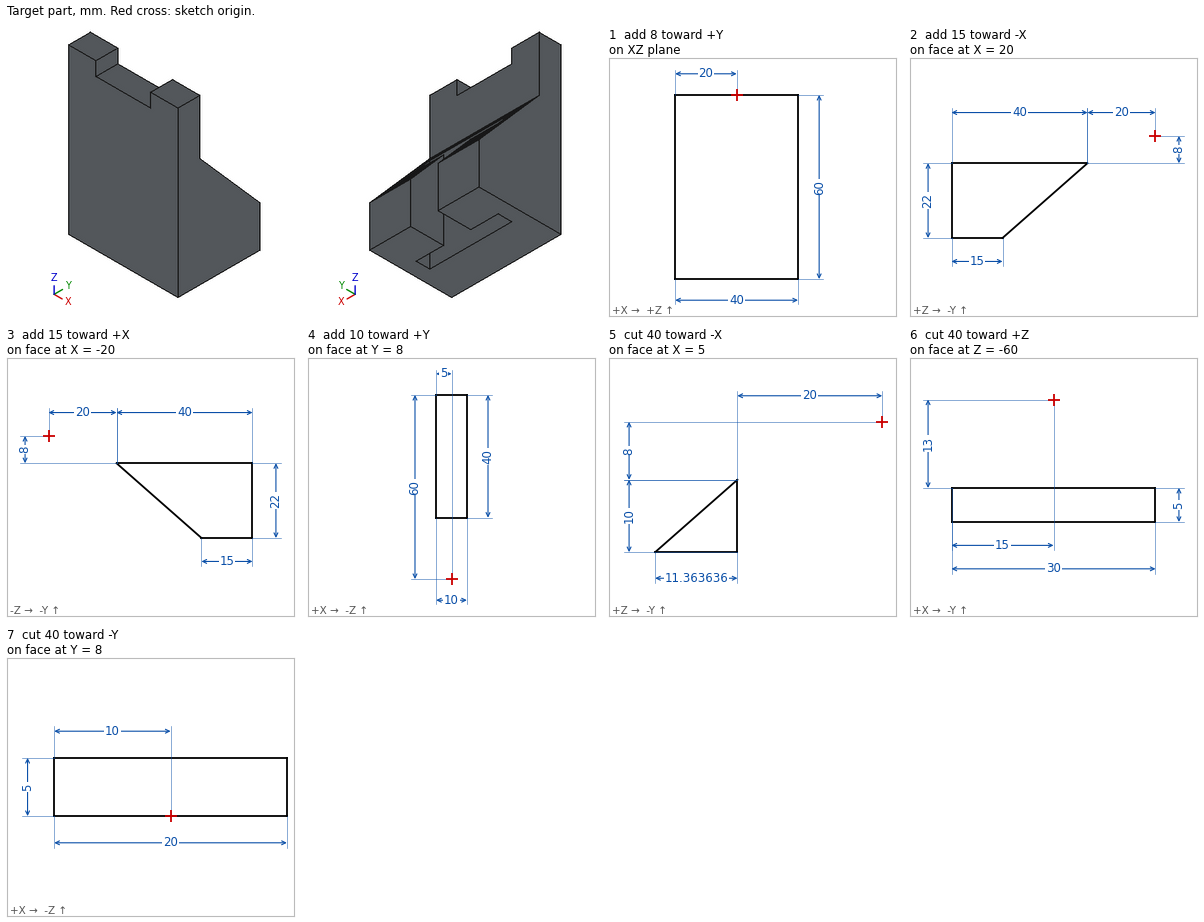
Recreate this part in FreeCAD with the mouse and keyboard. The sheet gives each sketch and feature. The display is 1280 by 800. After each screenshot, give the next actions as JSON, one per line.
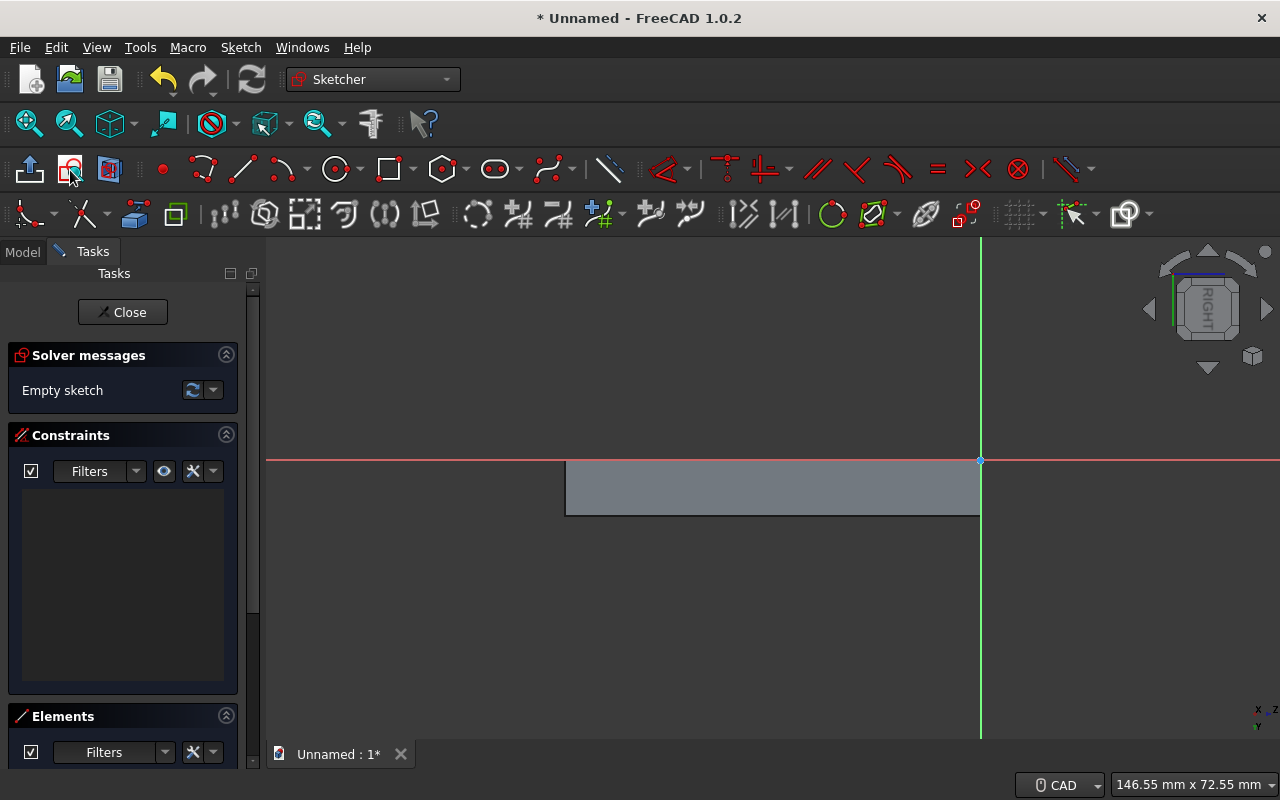
{"action": "scroll", "coordinate": [912, 711], "scroll_direction": "up", "scroll_amount": 2}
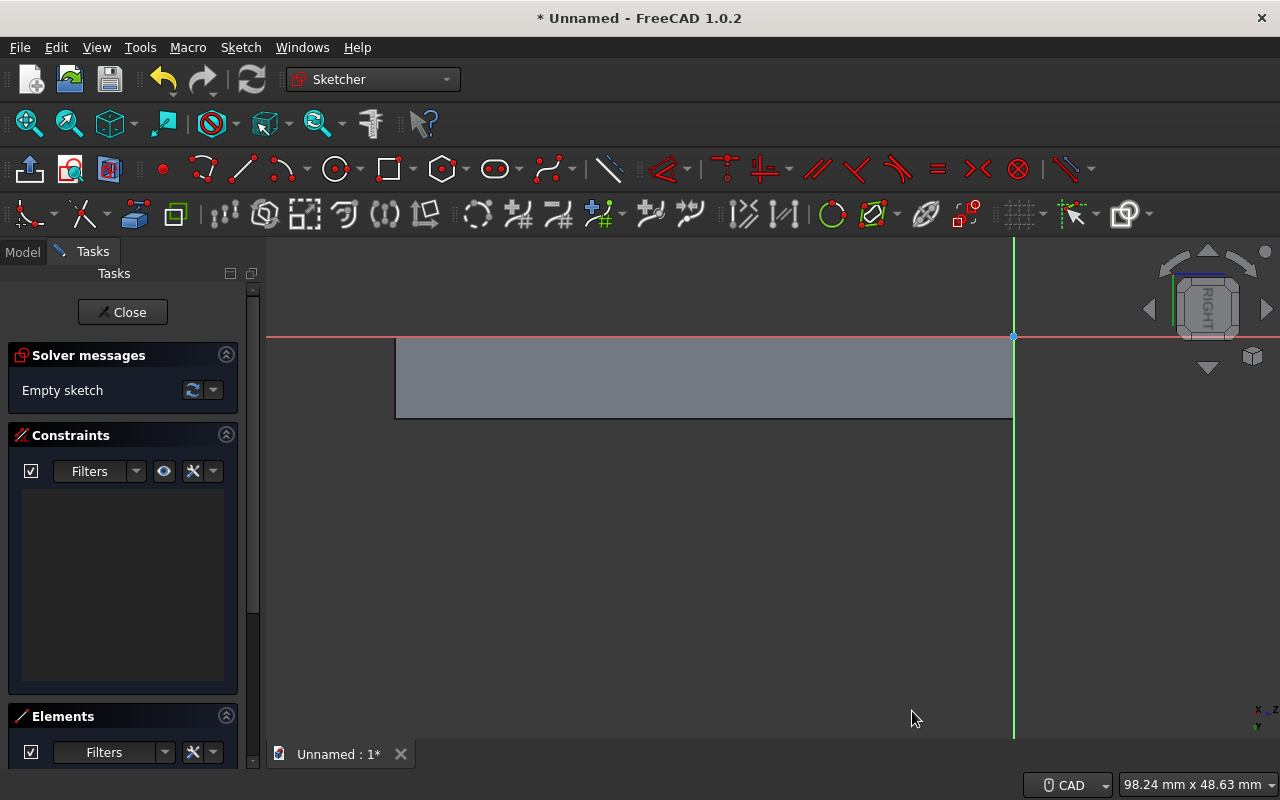
{"action": "left_click", "coordinate": [204, 170]}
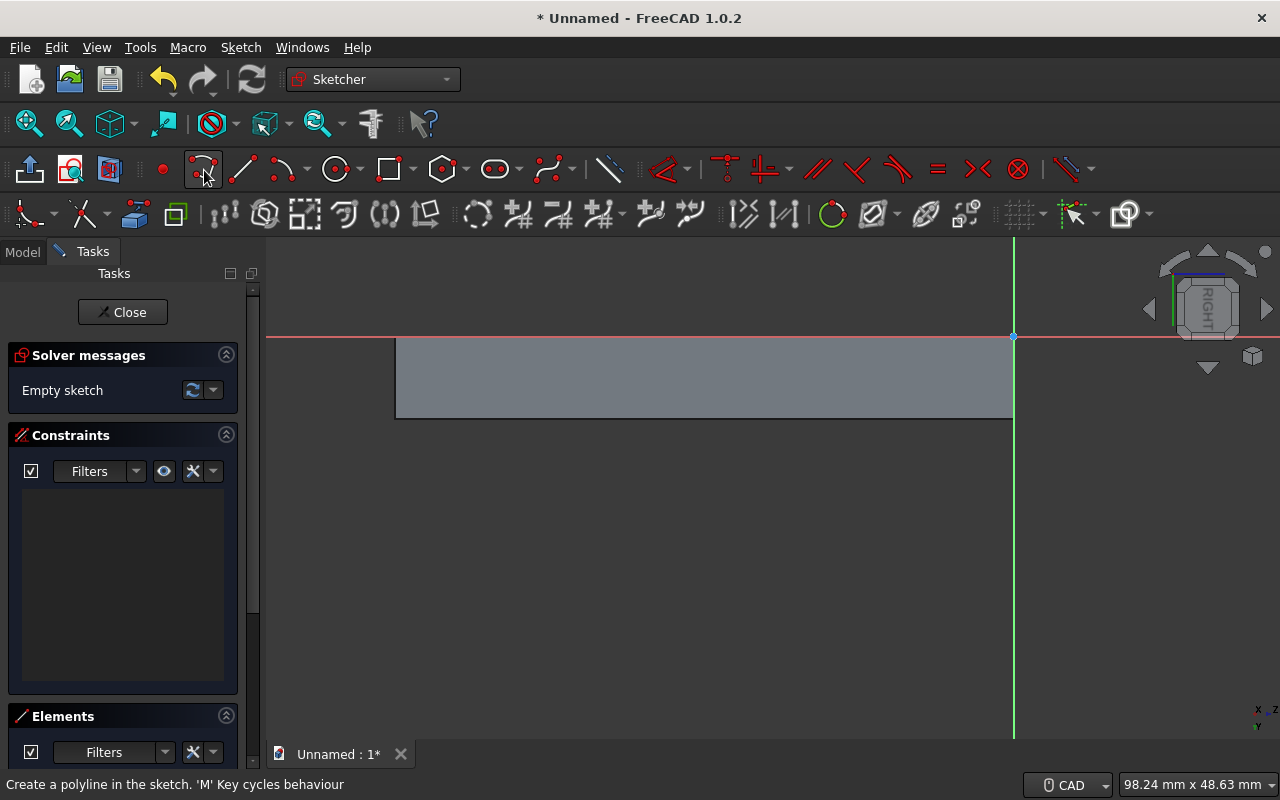
{"action": "left_click", "coordinate": [808, 419]}
{"action": "left_click", "coordinate": [395, 419]}
{"action": "left_click", "coordinate": [395, 646]}
{"action": "left_click", "coordinate": [549, 646]}
{"action": "left_click", "coordinate": [808, 420]}
{"action": "key", "text": "Escape"}
{"action": "key", "text": "Escape"}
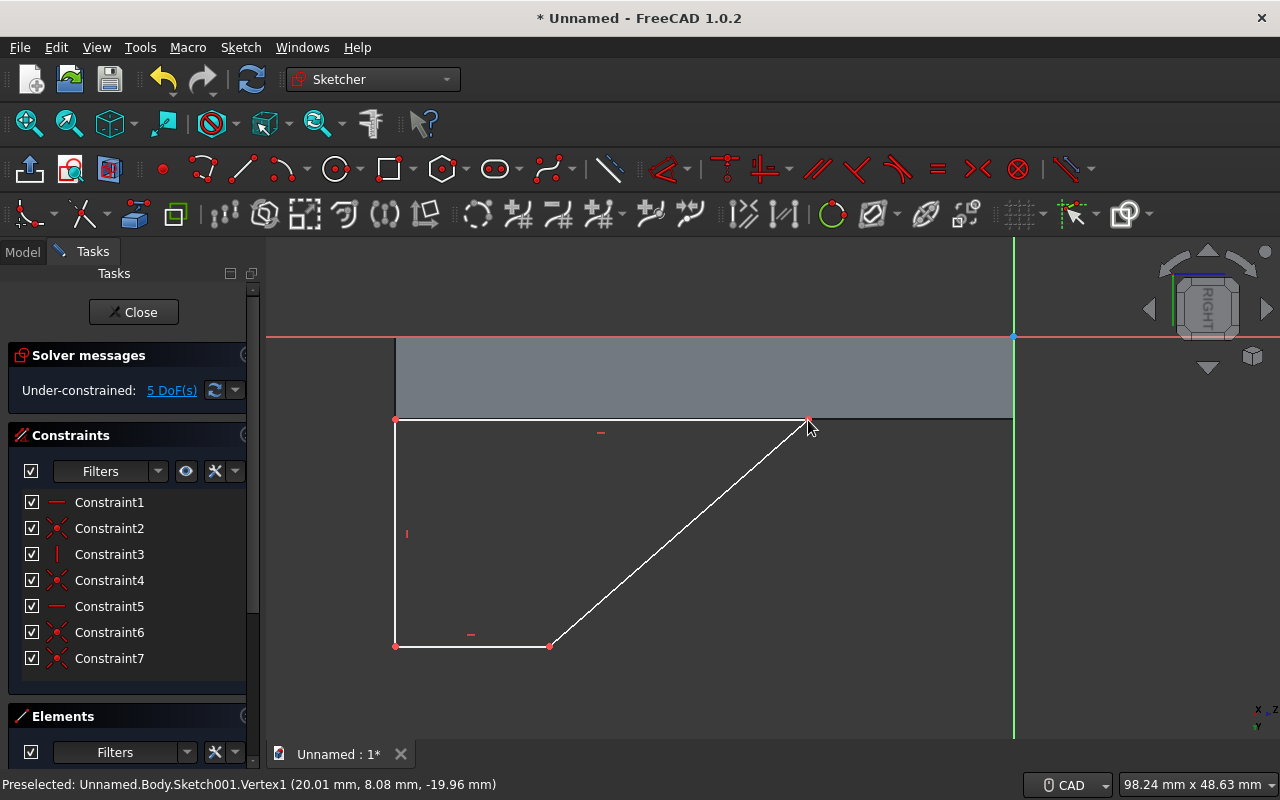
{"action": "left_click", "coordinate": [684, 420]}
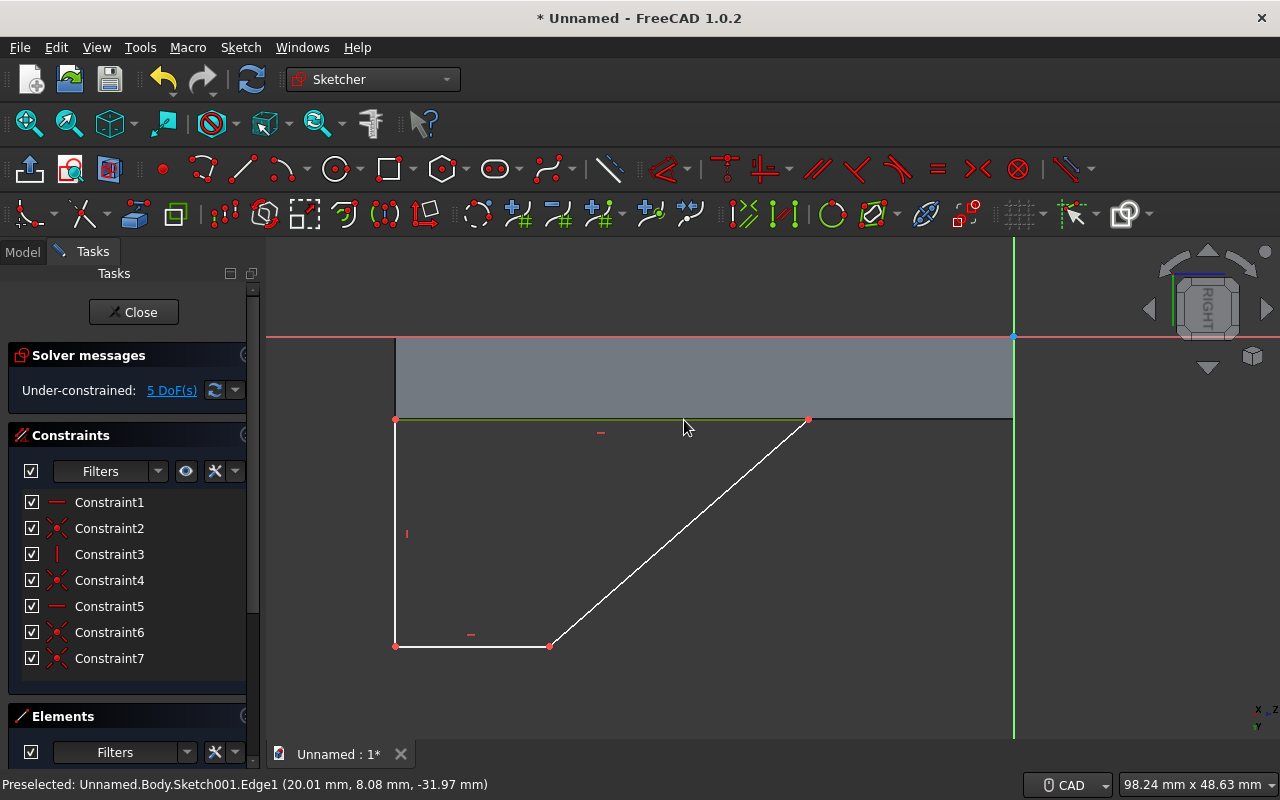
{"action": "key", "text": "l"}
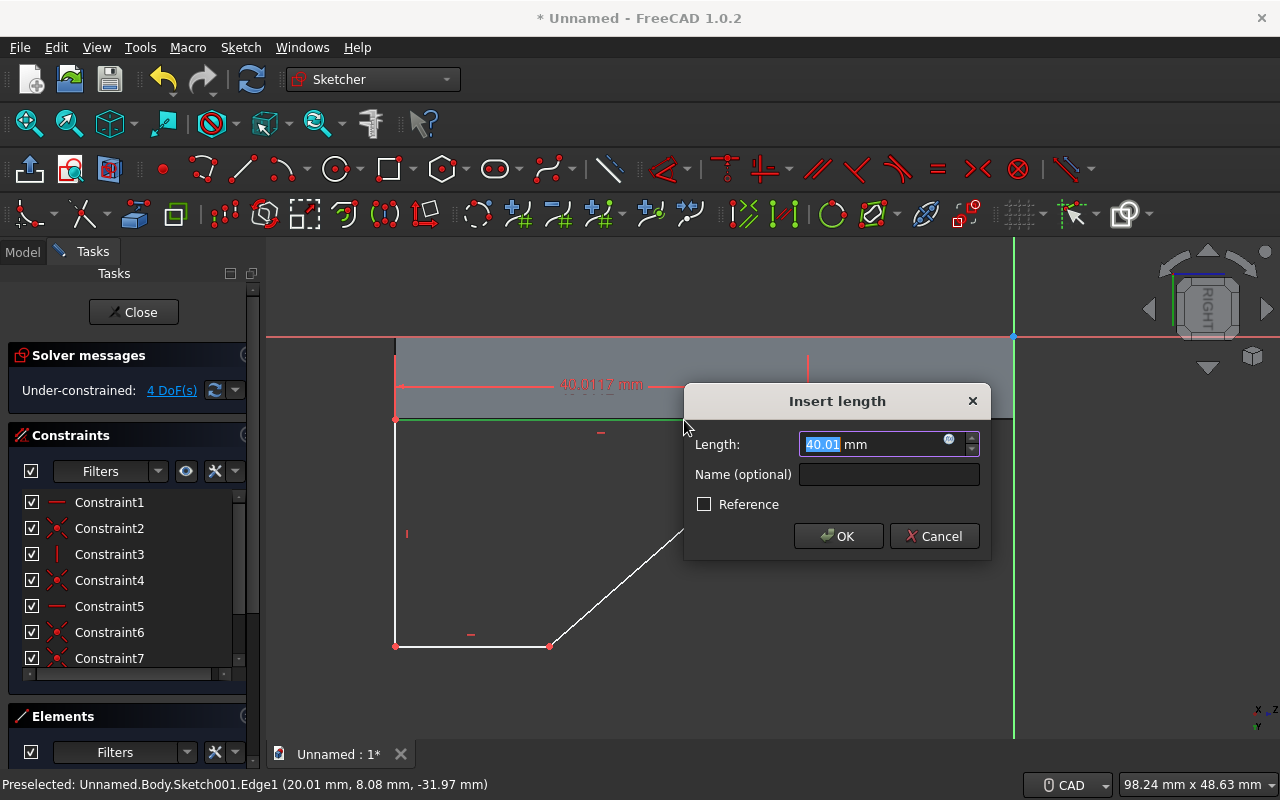
{"action": "type", "text": "40"}
{"action": "key", "text": "Return"}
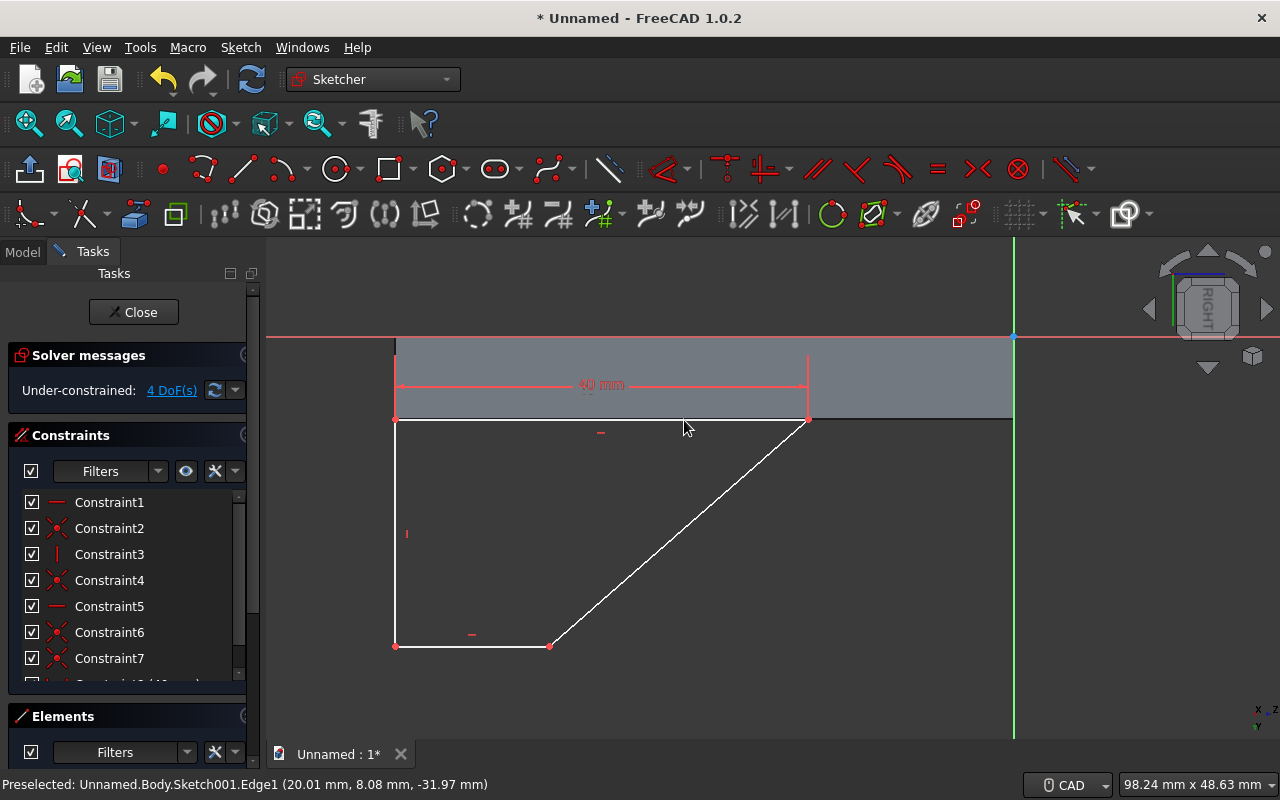
{"action": "left_click", "coordinate": [395, 488]}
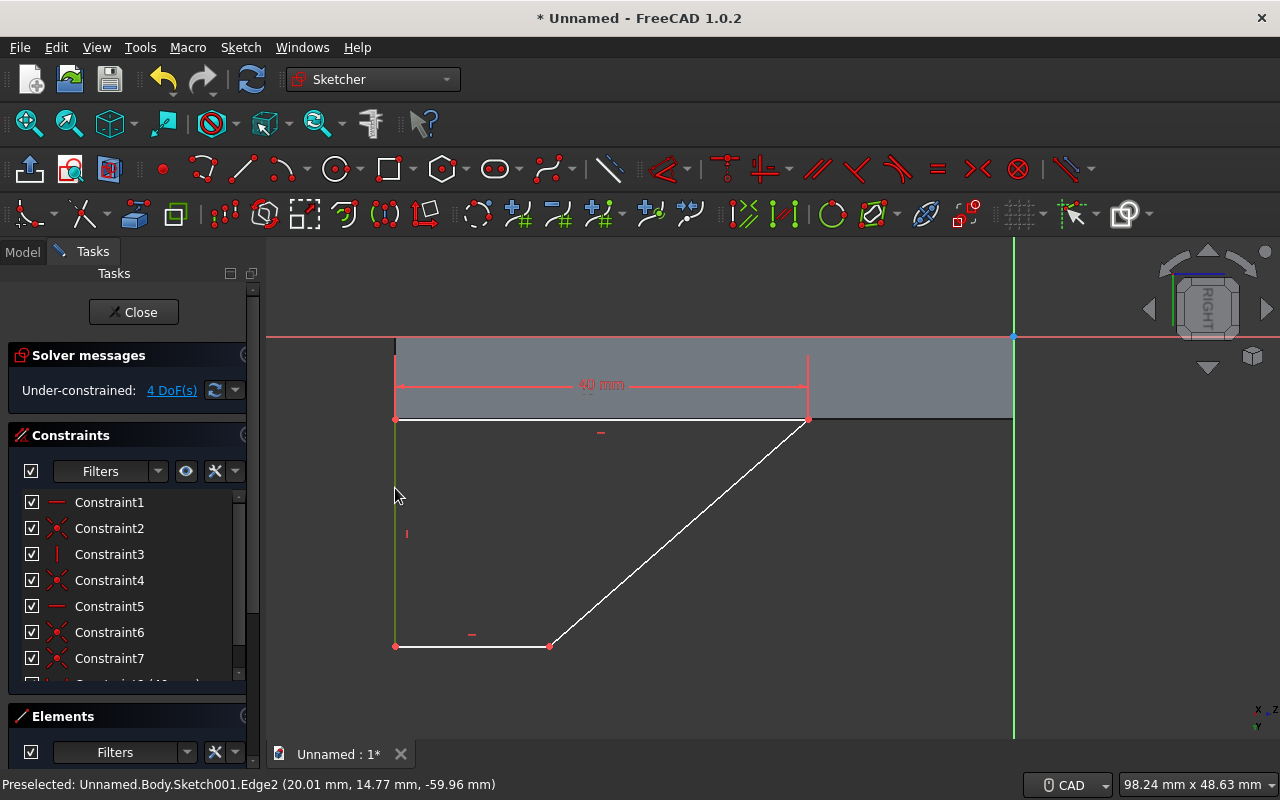
{"action": "left_click", "coordinate": [690, 170]}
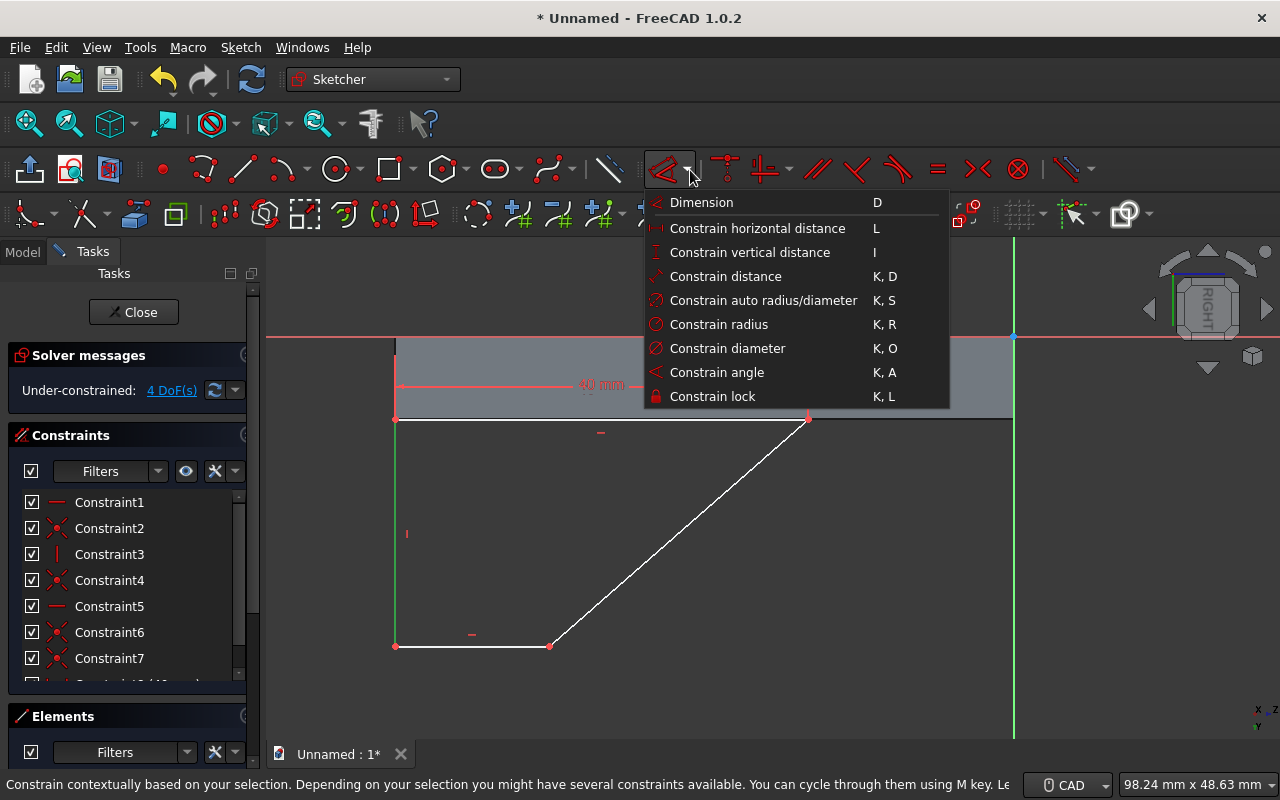
{"action": "left_click", "coordinate": [797, 252]}